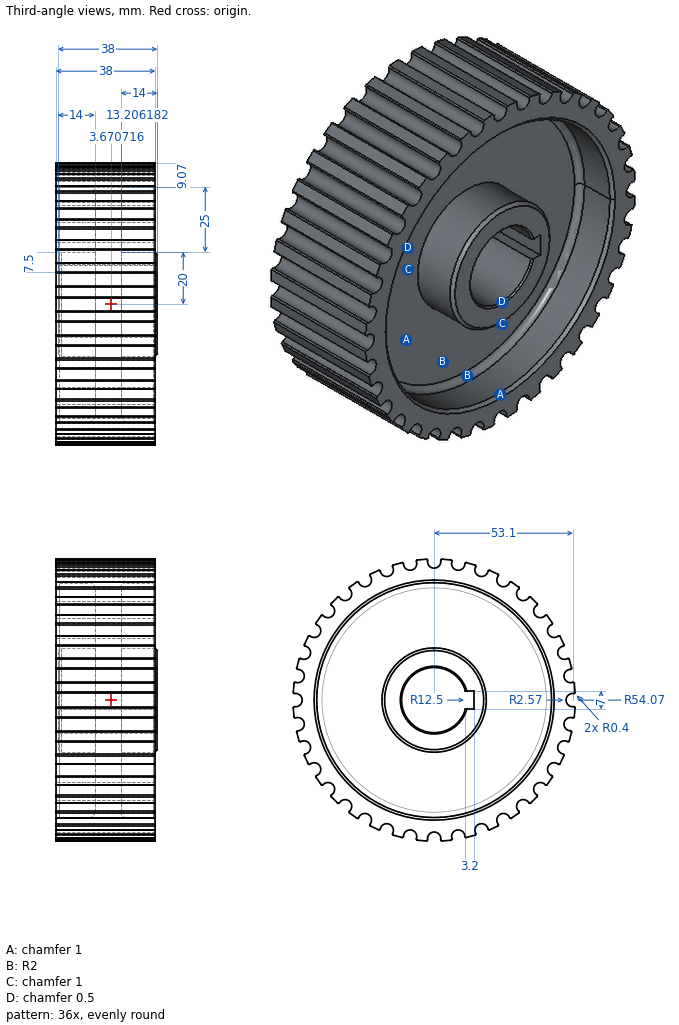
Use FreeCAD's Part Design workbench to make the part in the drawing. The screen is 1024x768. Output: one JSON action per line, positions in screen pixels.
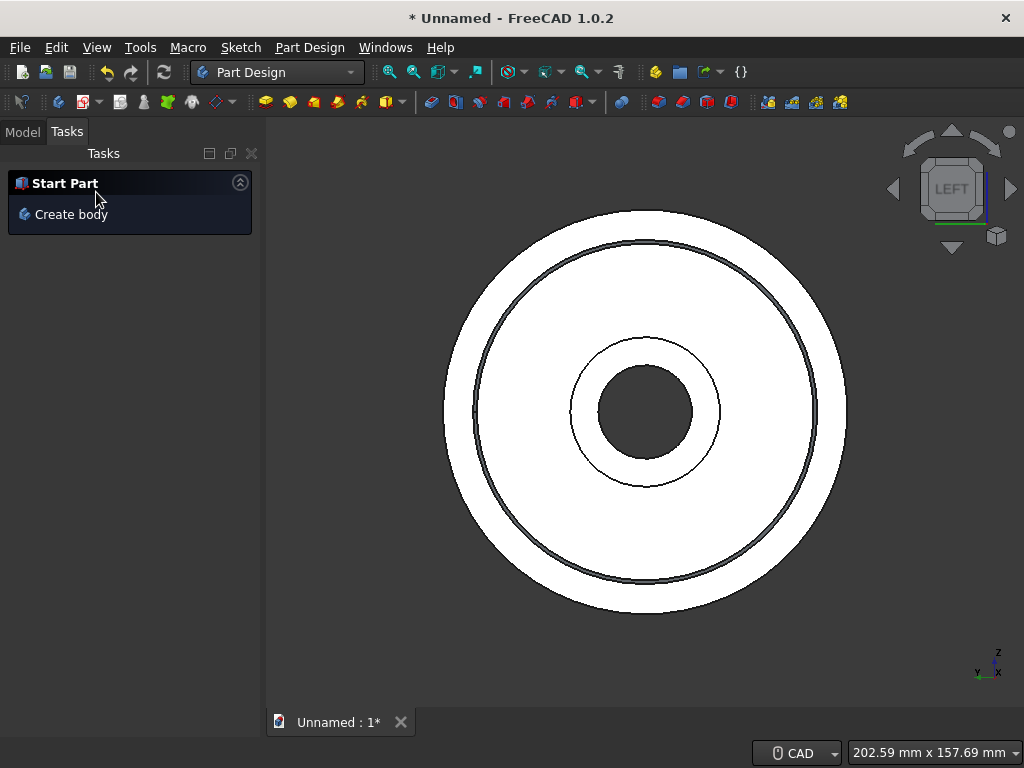
{"action": "key", "text": "v 3"}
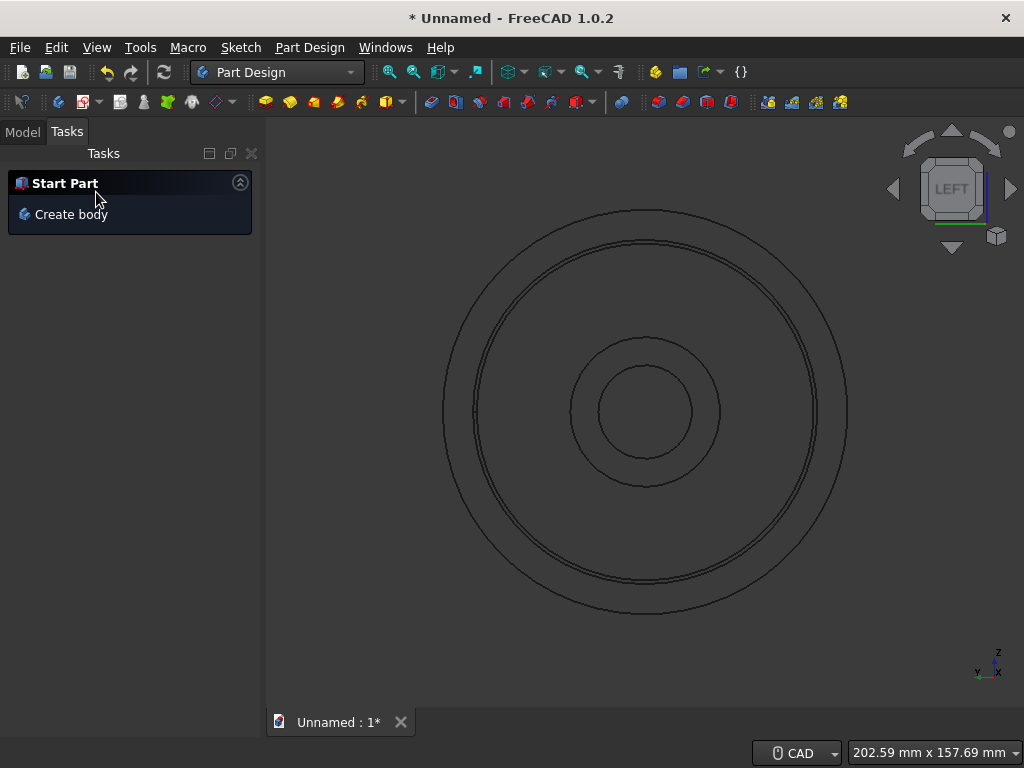
{"action": "key", "text": "0"}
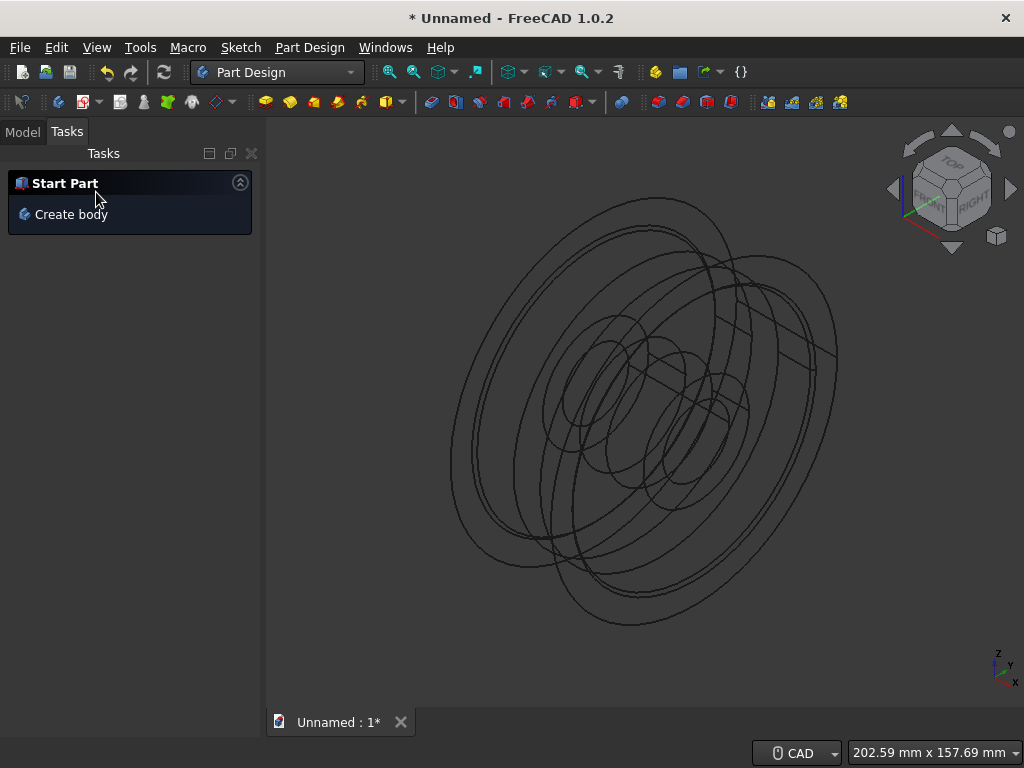
{"action": "left_click", "coordinate": [540, 488]}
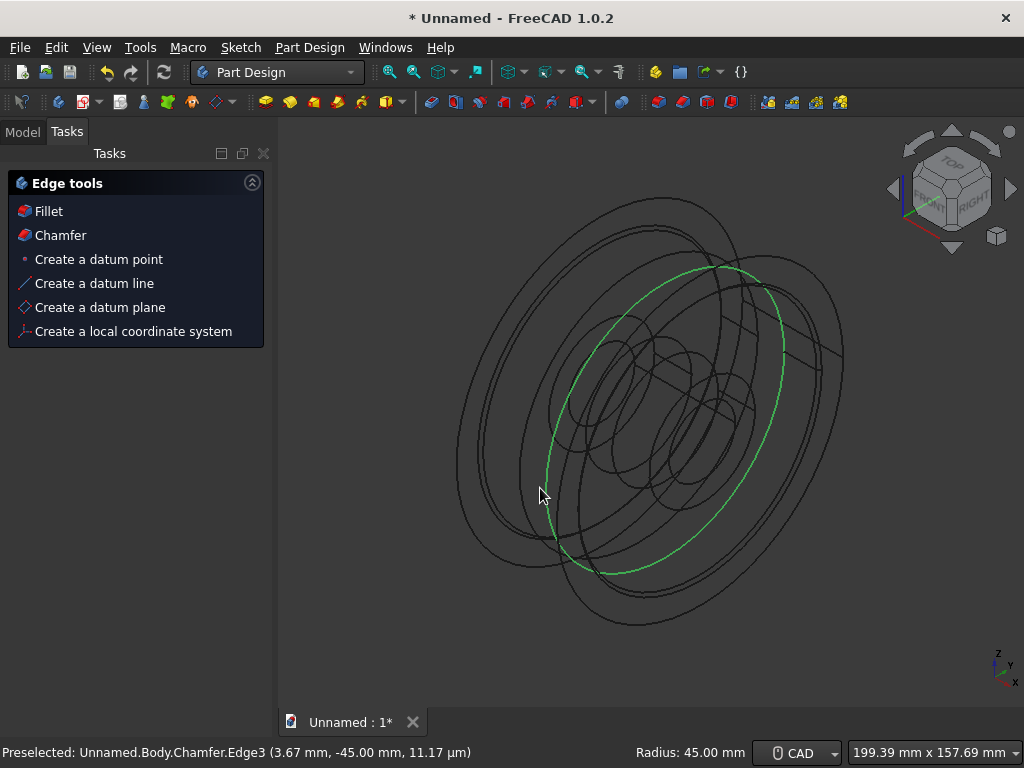
{"action": "left_click", "coordinate": [520, 473], "text": "ctrl"}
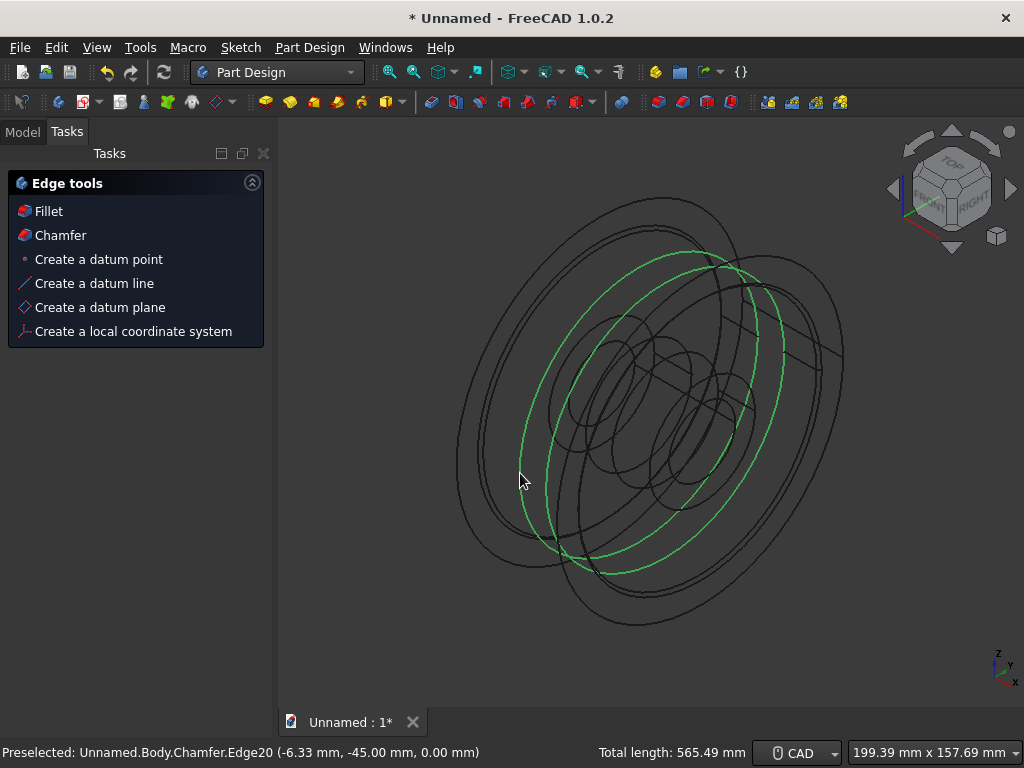
{"action": "key", "text": "v 1"}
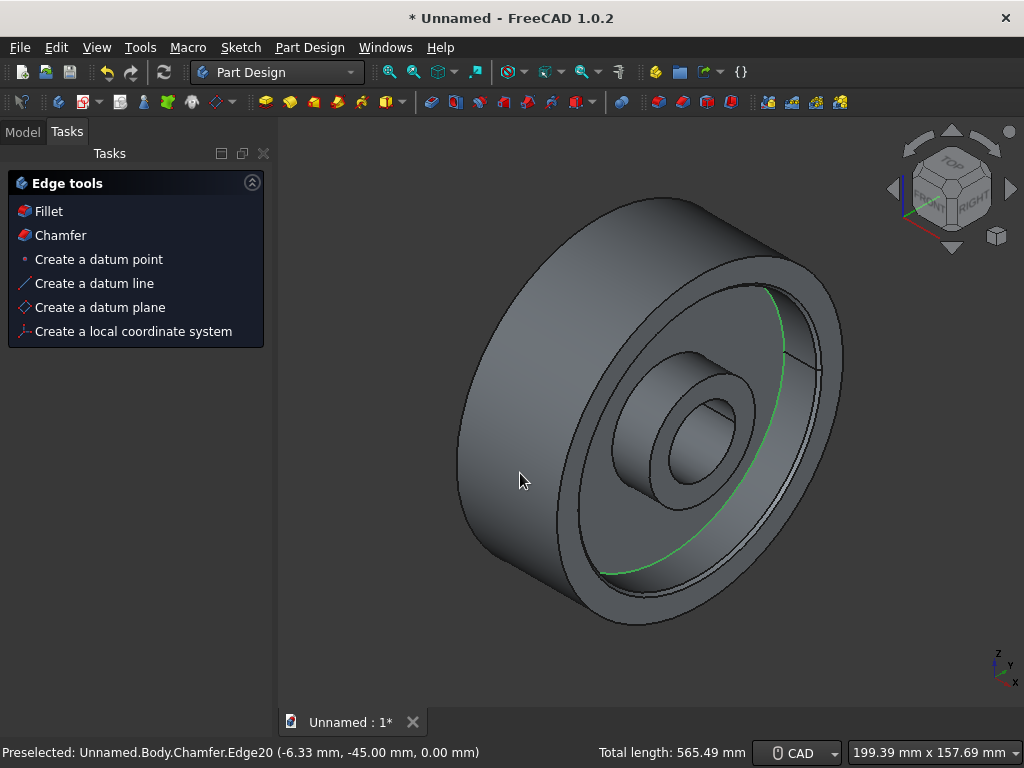
{"action": "left_click", "coordinate": [660, 102]}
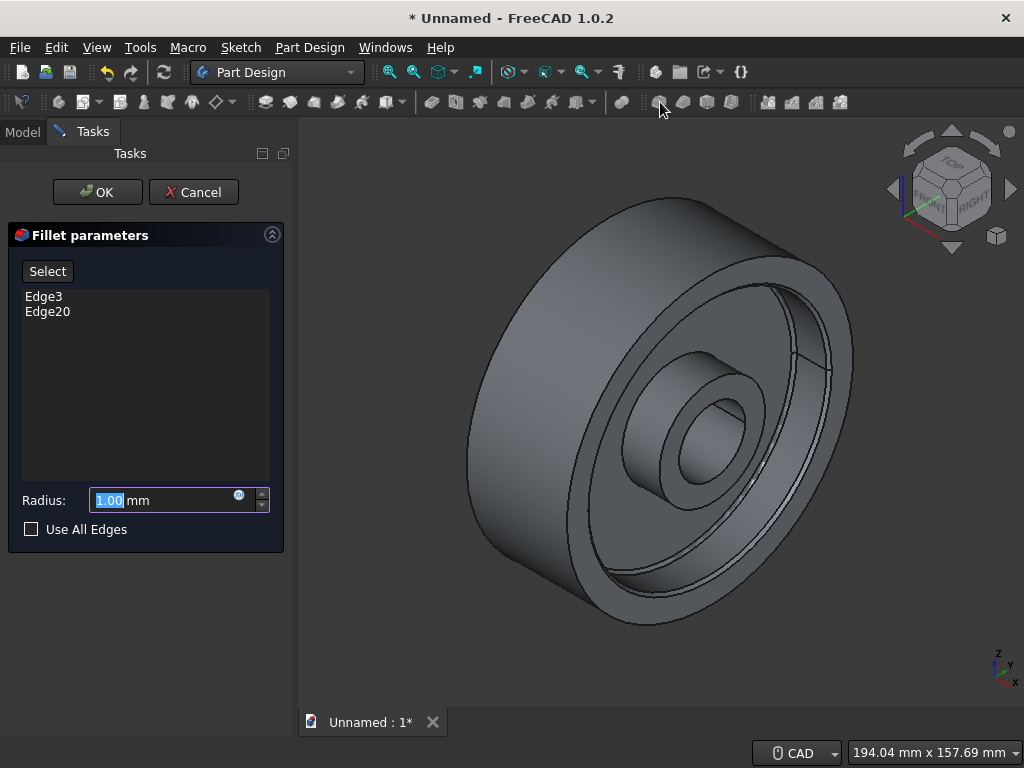
{"action": "type", "text": "2"}
{"action": "key", "text": "Tab"}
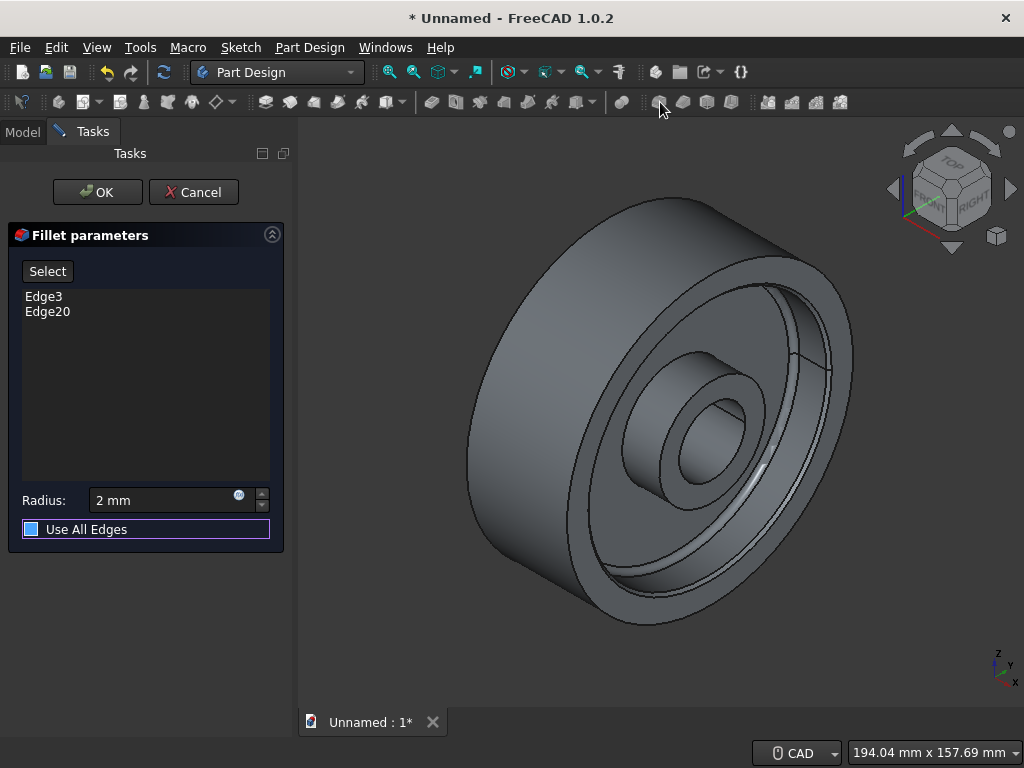
{"action": "left_click", "coordinate": [98, 192]}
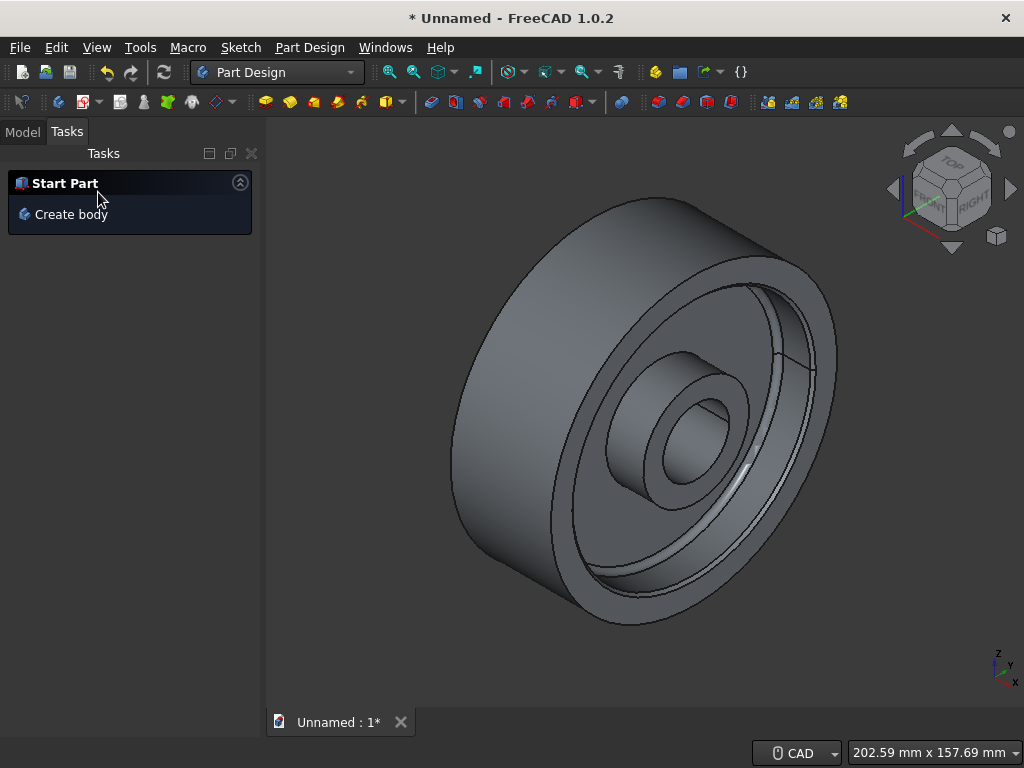
{"action": "left_click", "coordinate": [643, 471]}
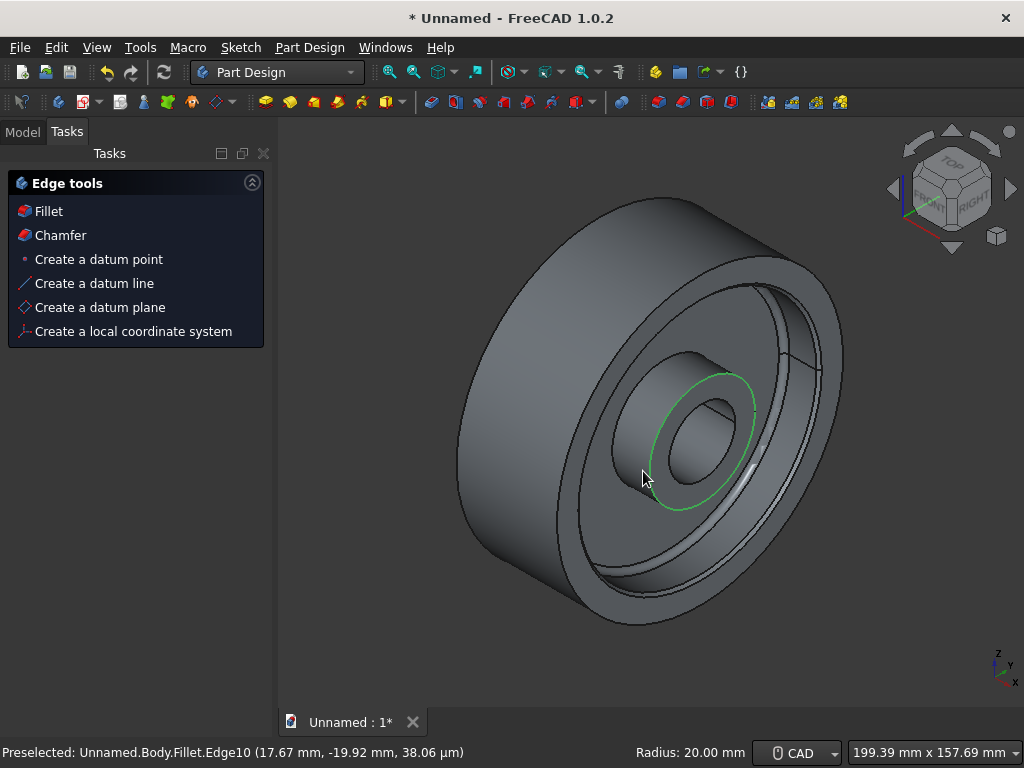
{"action": "key", "text": "2"}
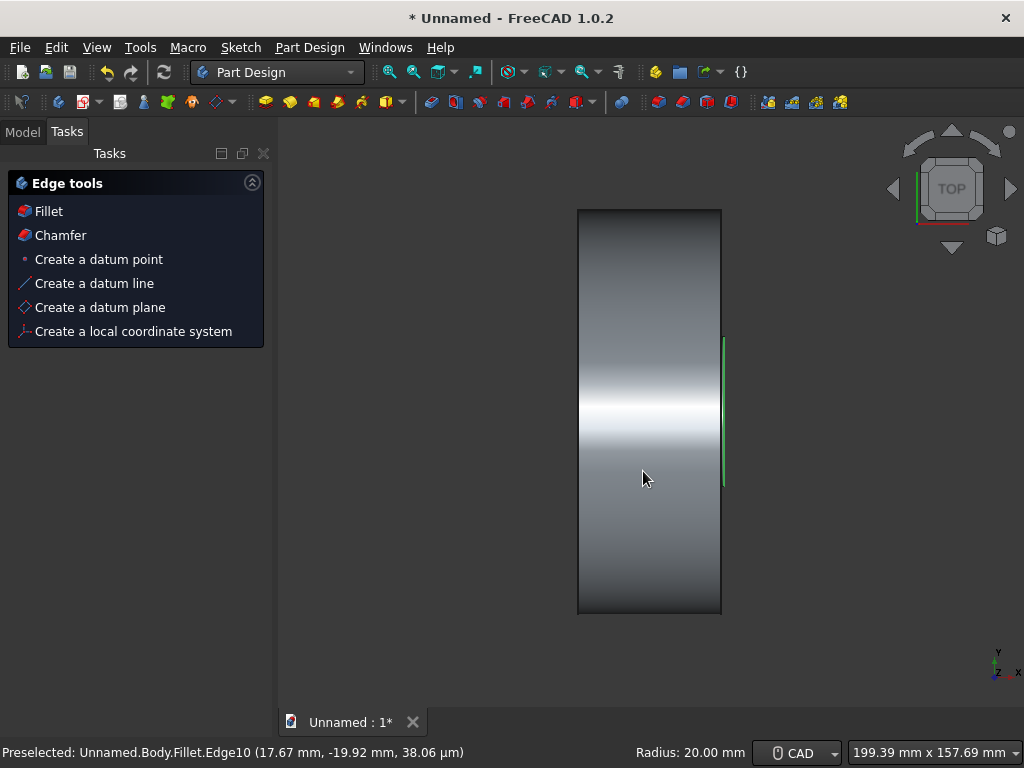
{"action": "key", "text": "0"}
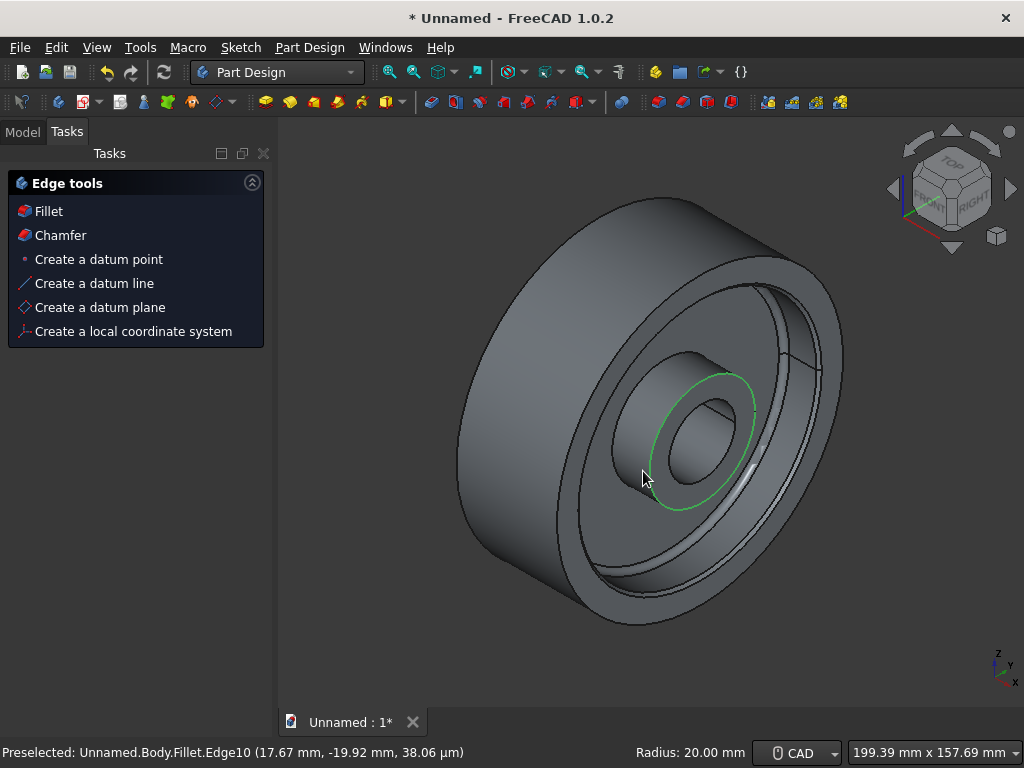
{"action": "key", "text": "1"}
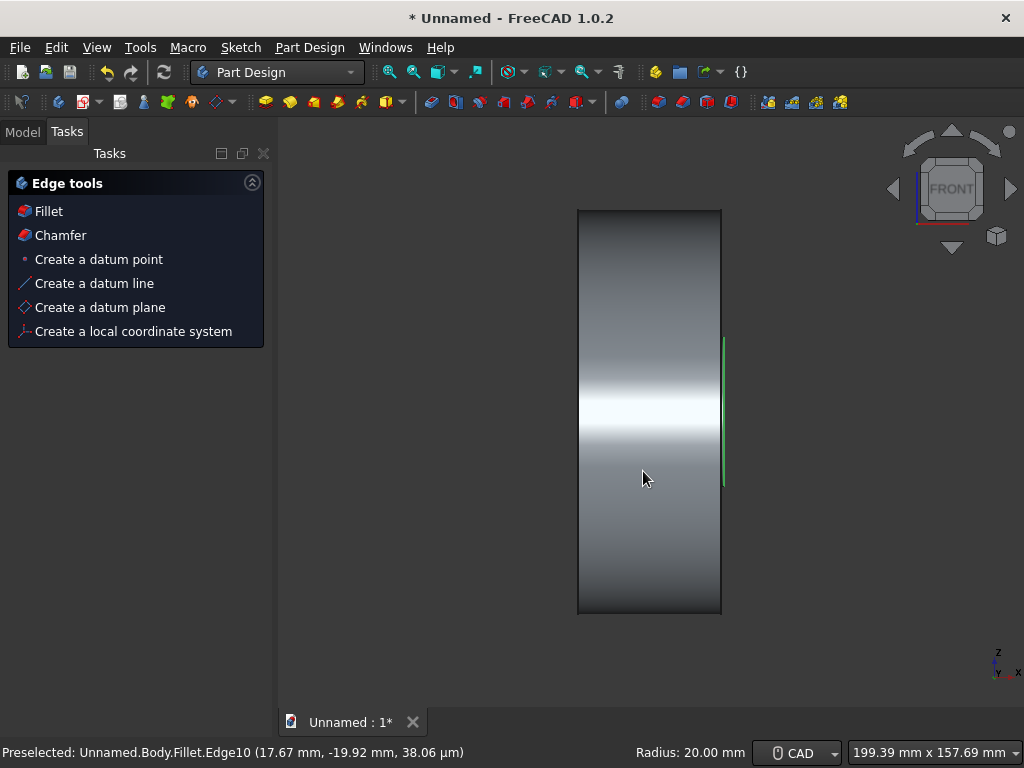
{"action": "key", "text": "3"}